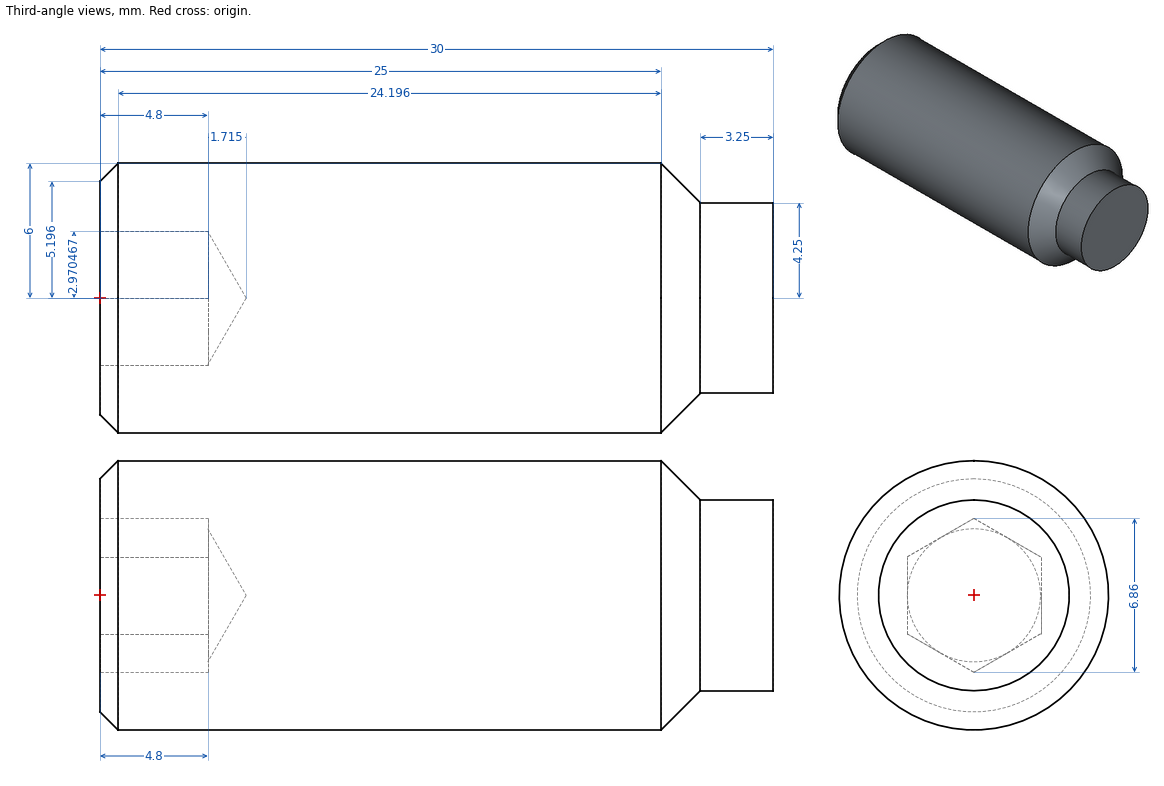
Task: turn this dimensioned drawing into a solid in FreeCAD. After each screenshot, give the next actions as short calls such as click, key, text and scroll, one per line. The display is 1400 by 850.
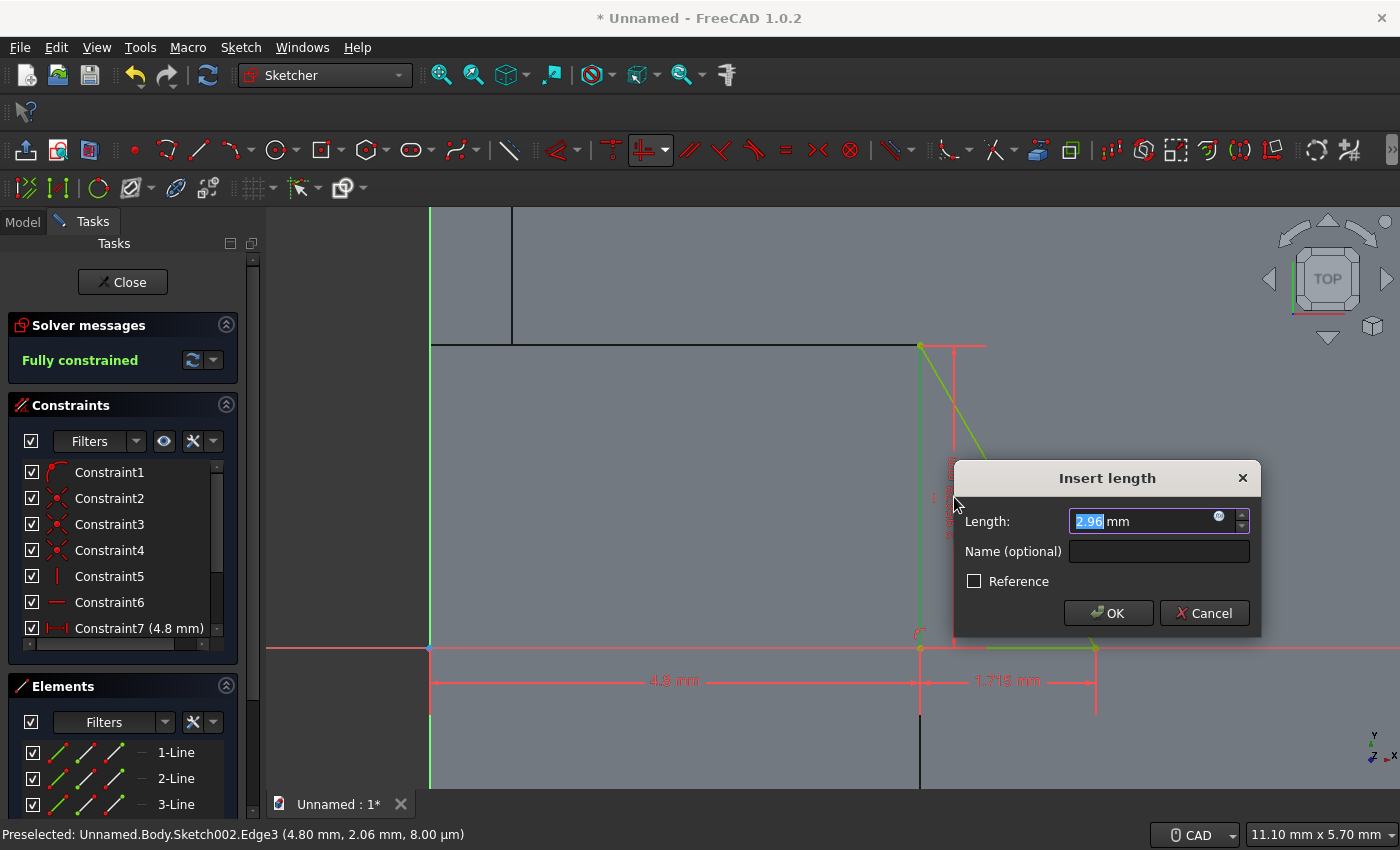
text(2.970467)
key(Return)
key(Escape)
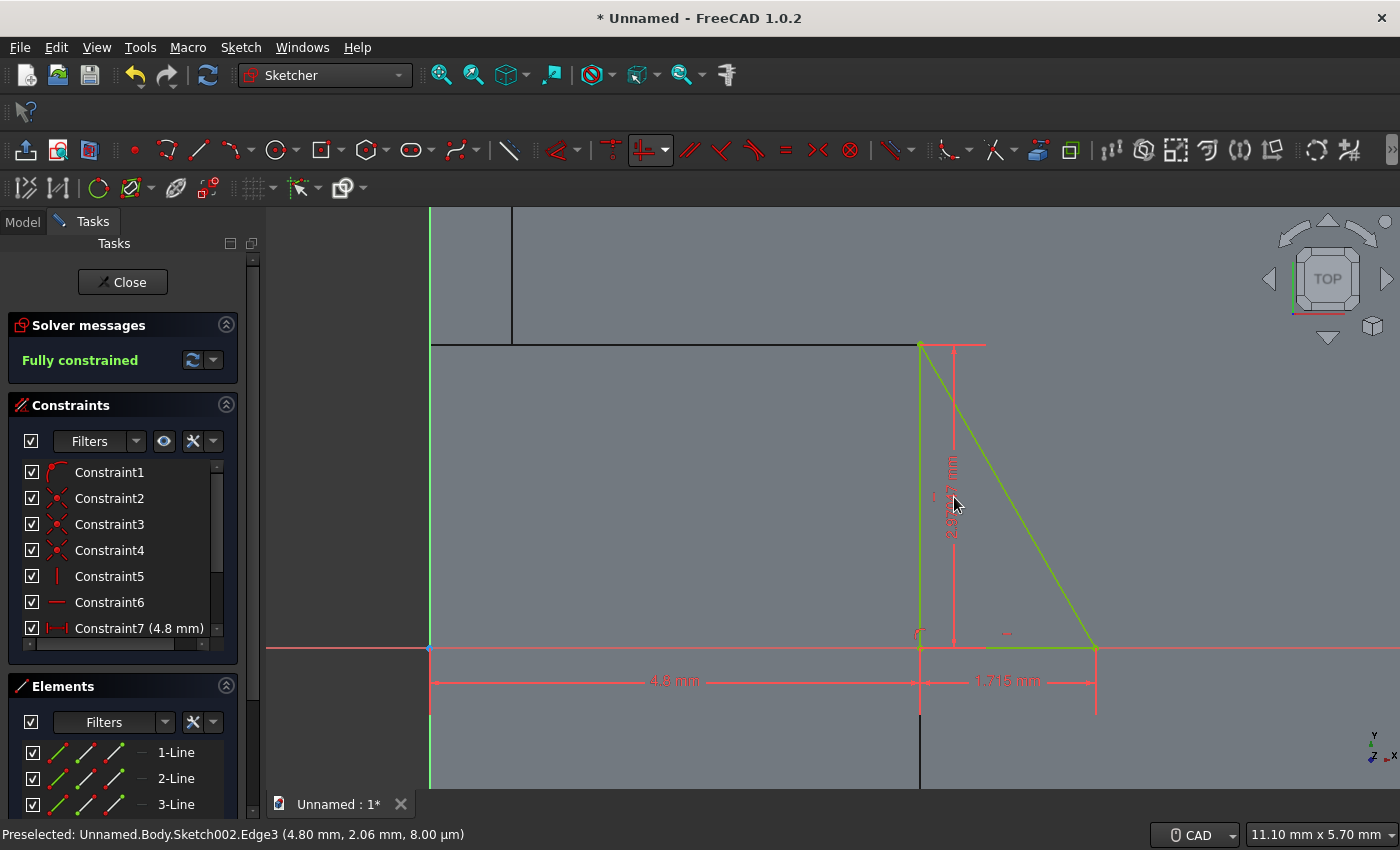
click(123, 282)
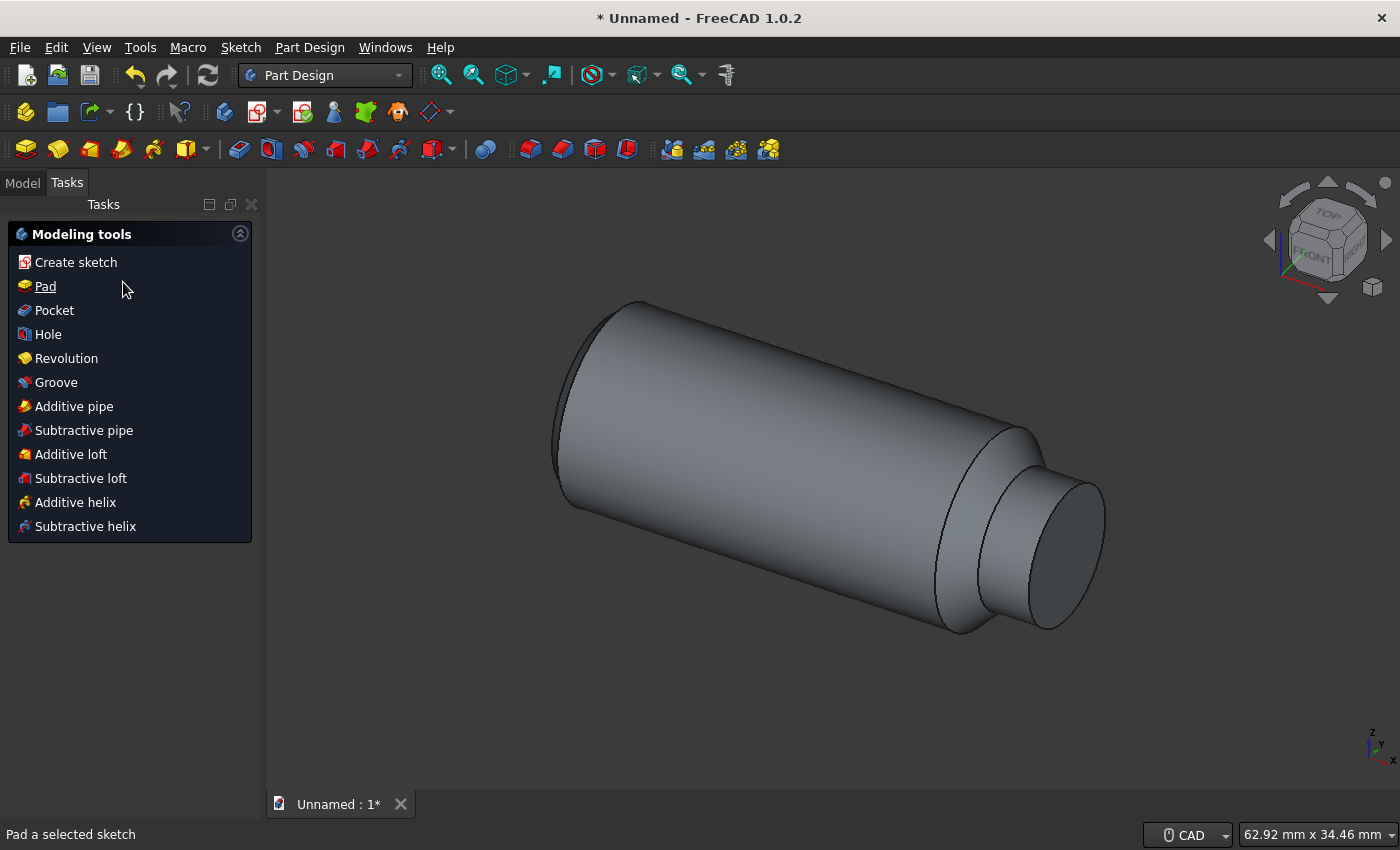
click(304, 150)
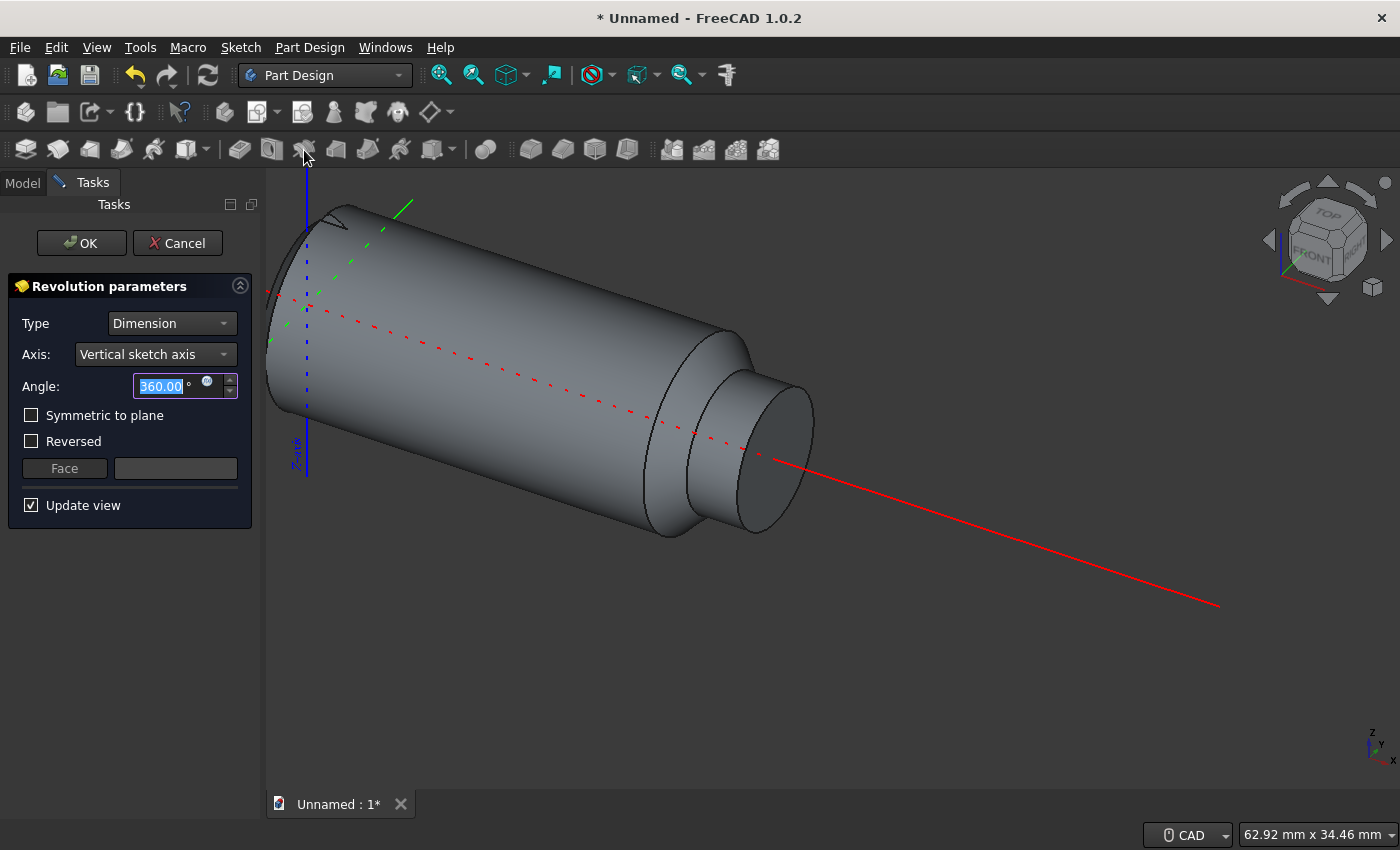
click(156, 354)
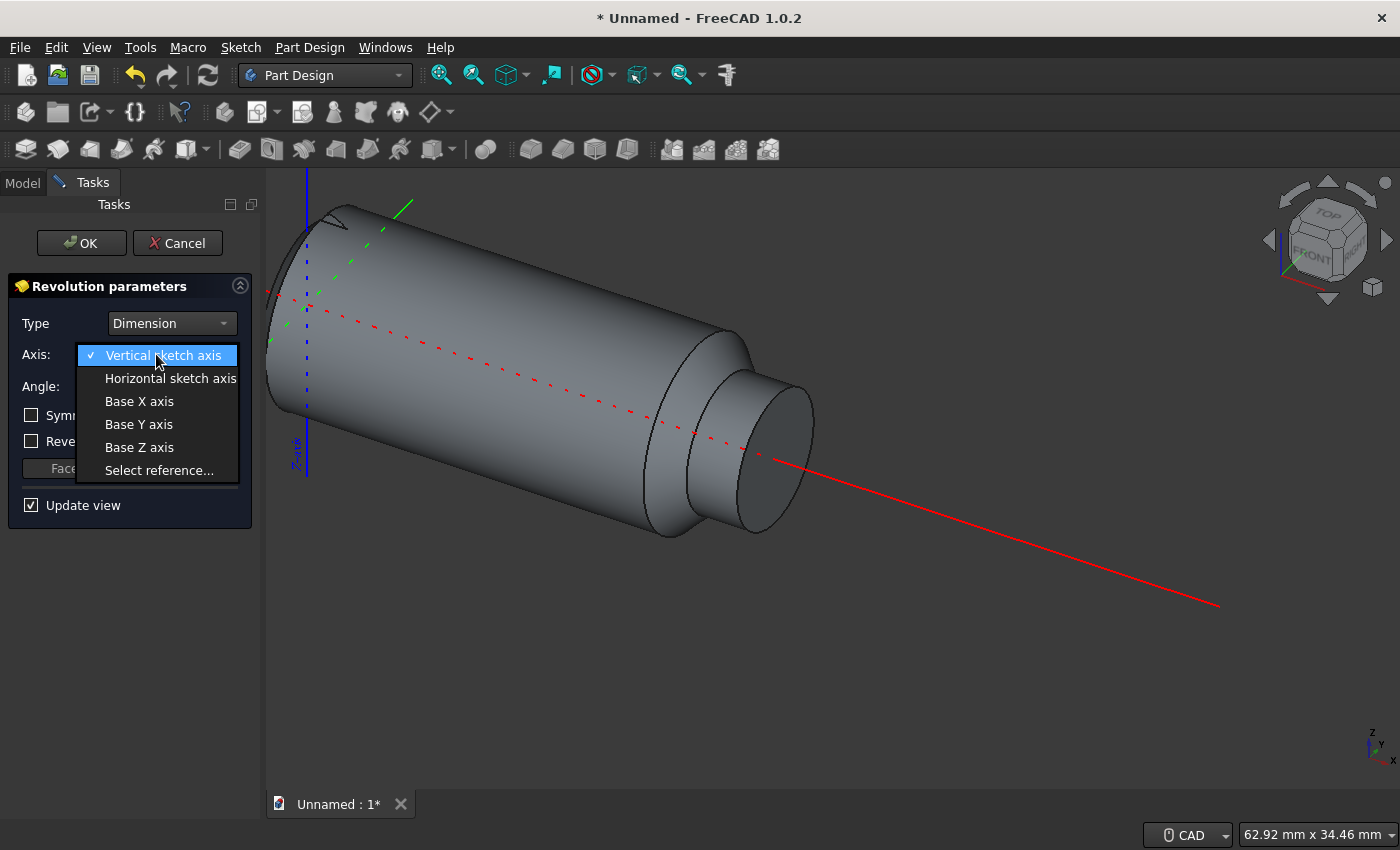
click(156, 378)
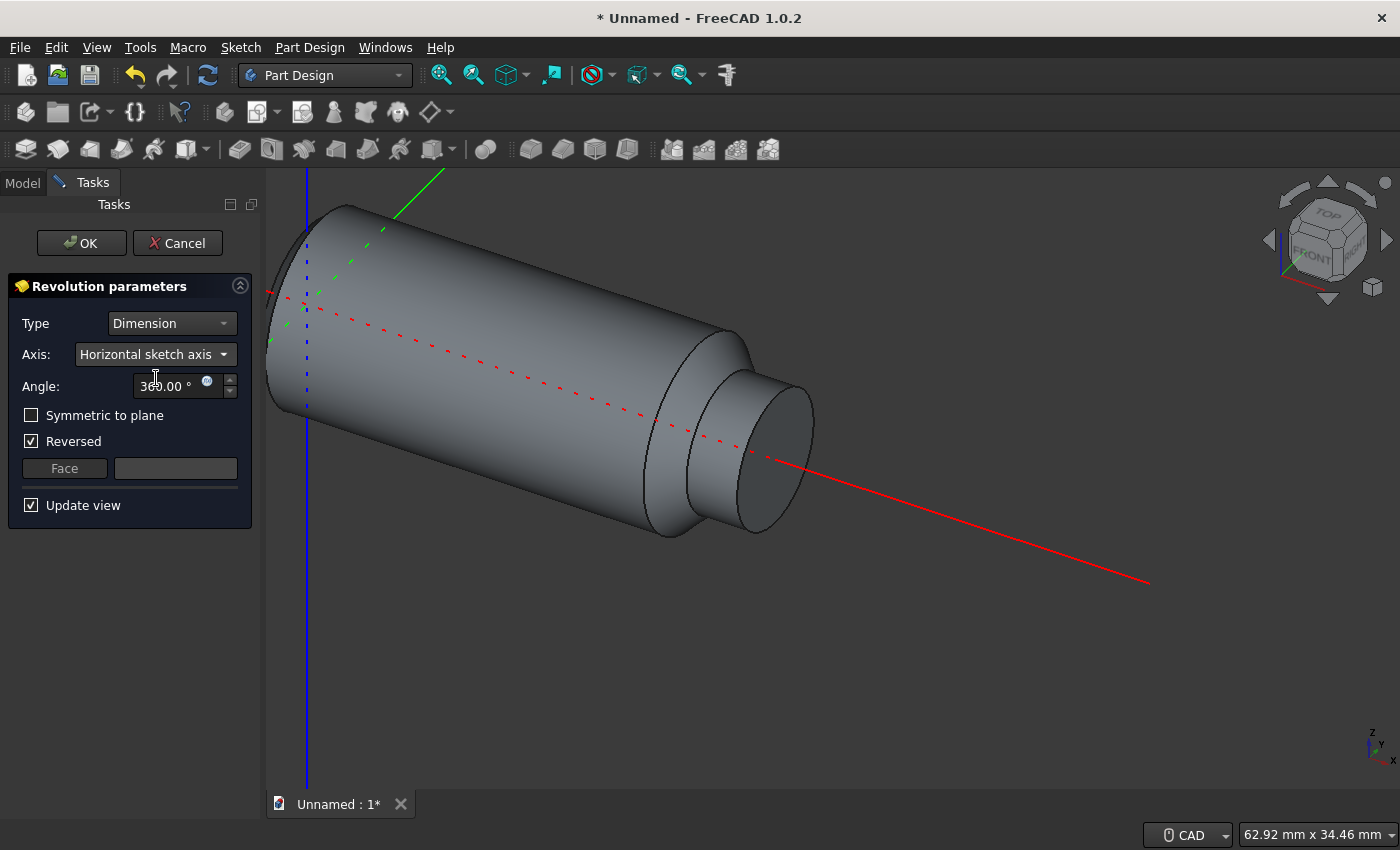
click(82, 243)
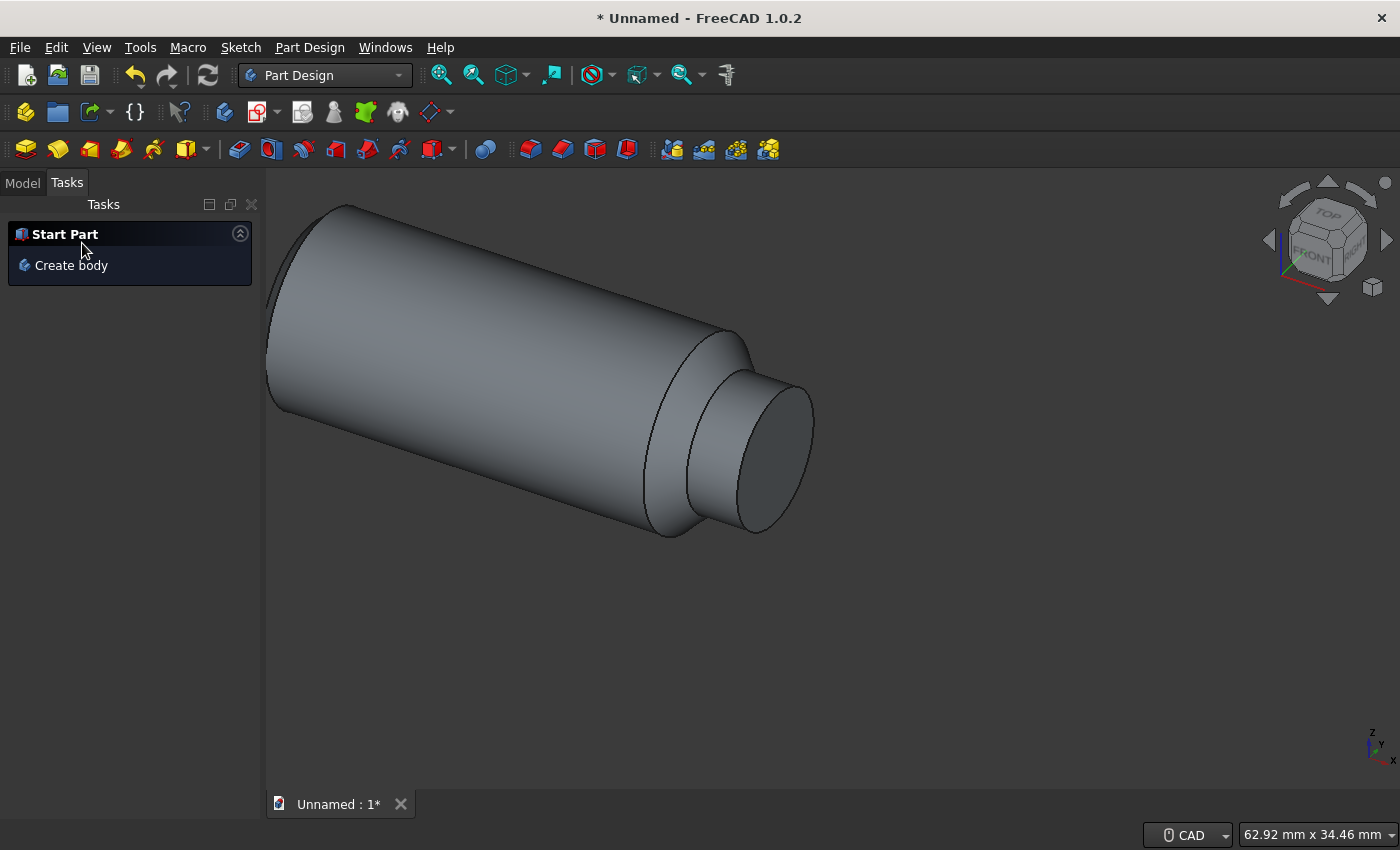
key(0)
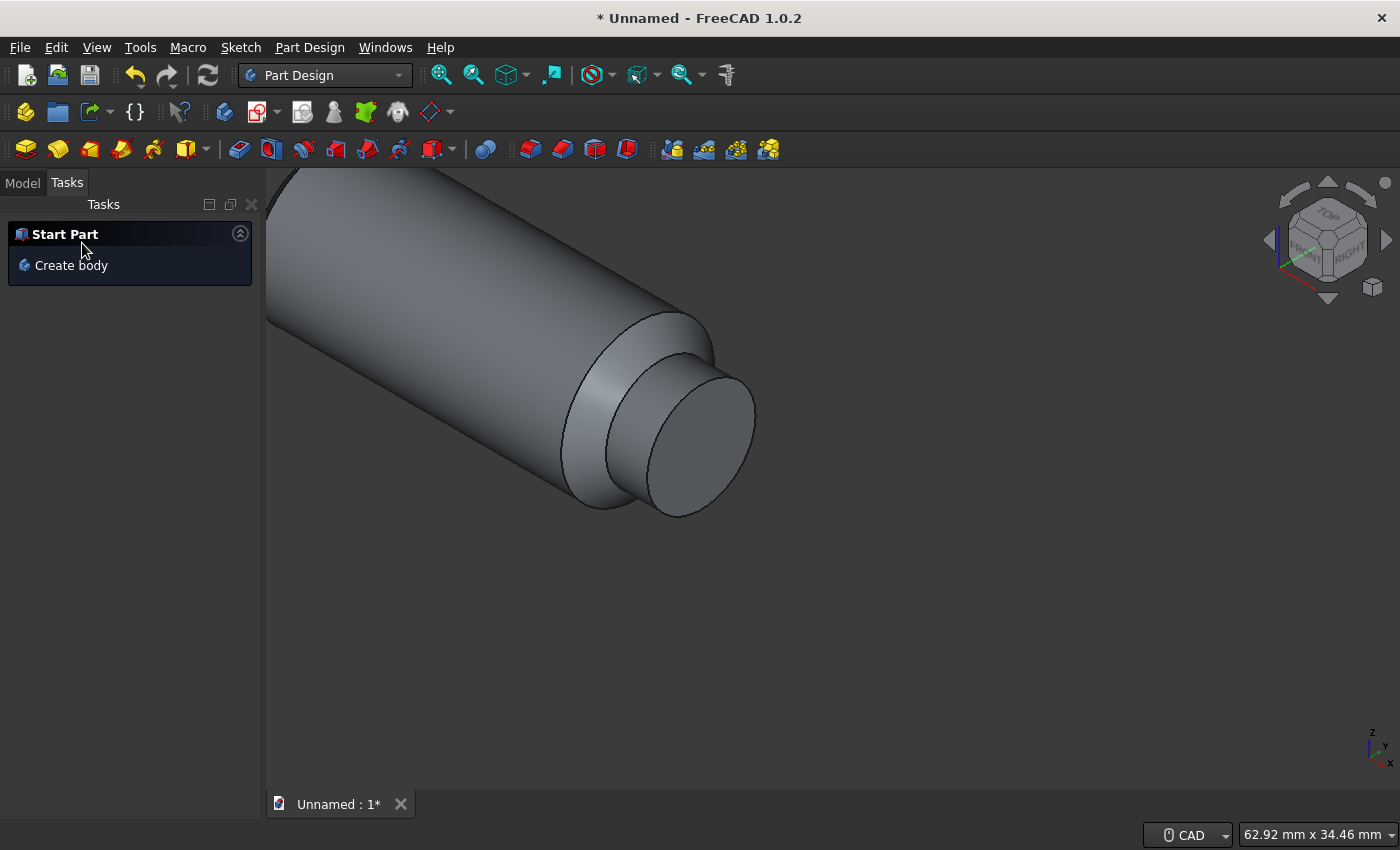
click(442, 76)